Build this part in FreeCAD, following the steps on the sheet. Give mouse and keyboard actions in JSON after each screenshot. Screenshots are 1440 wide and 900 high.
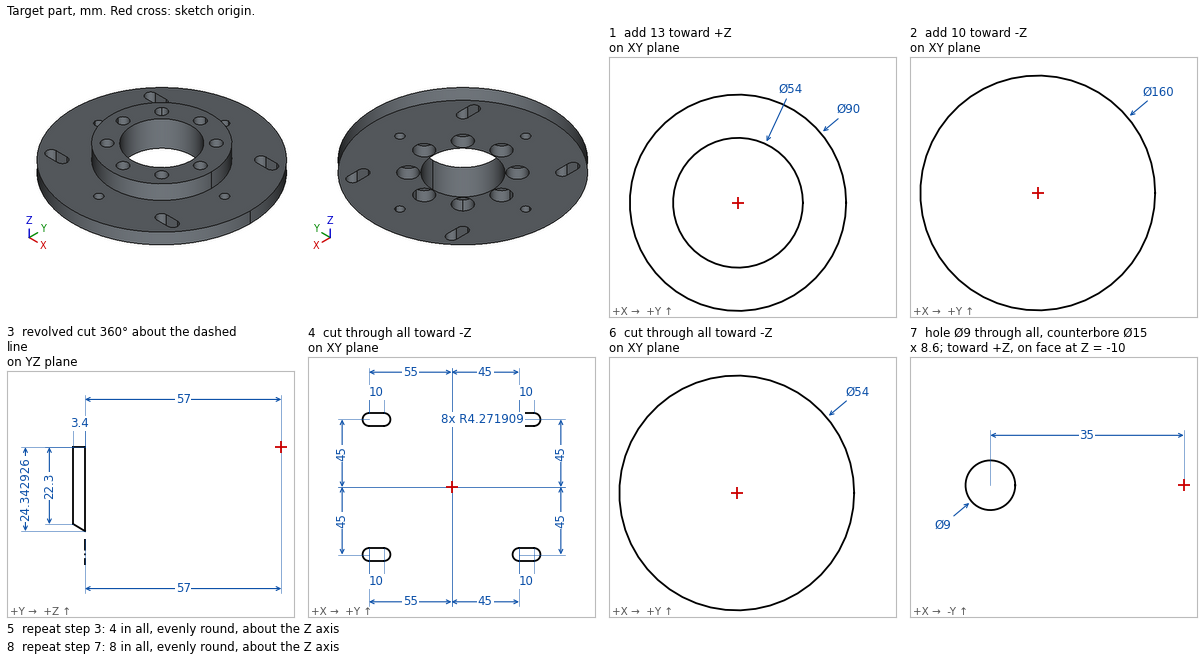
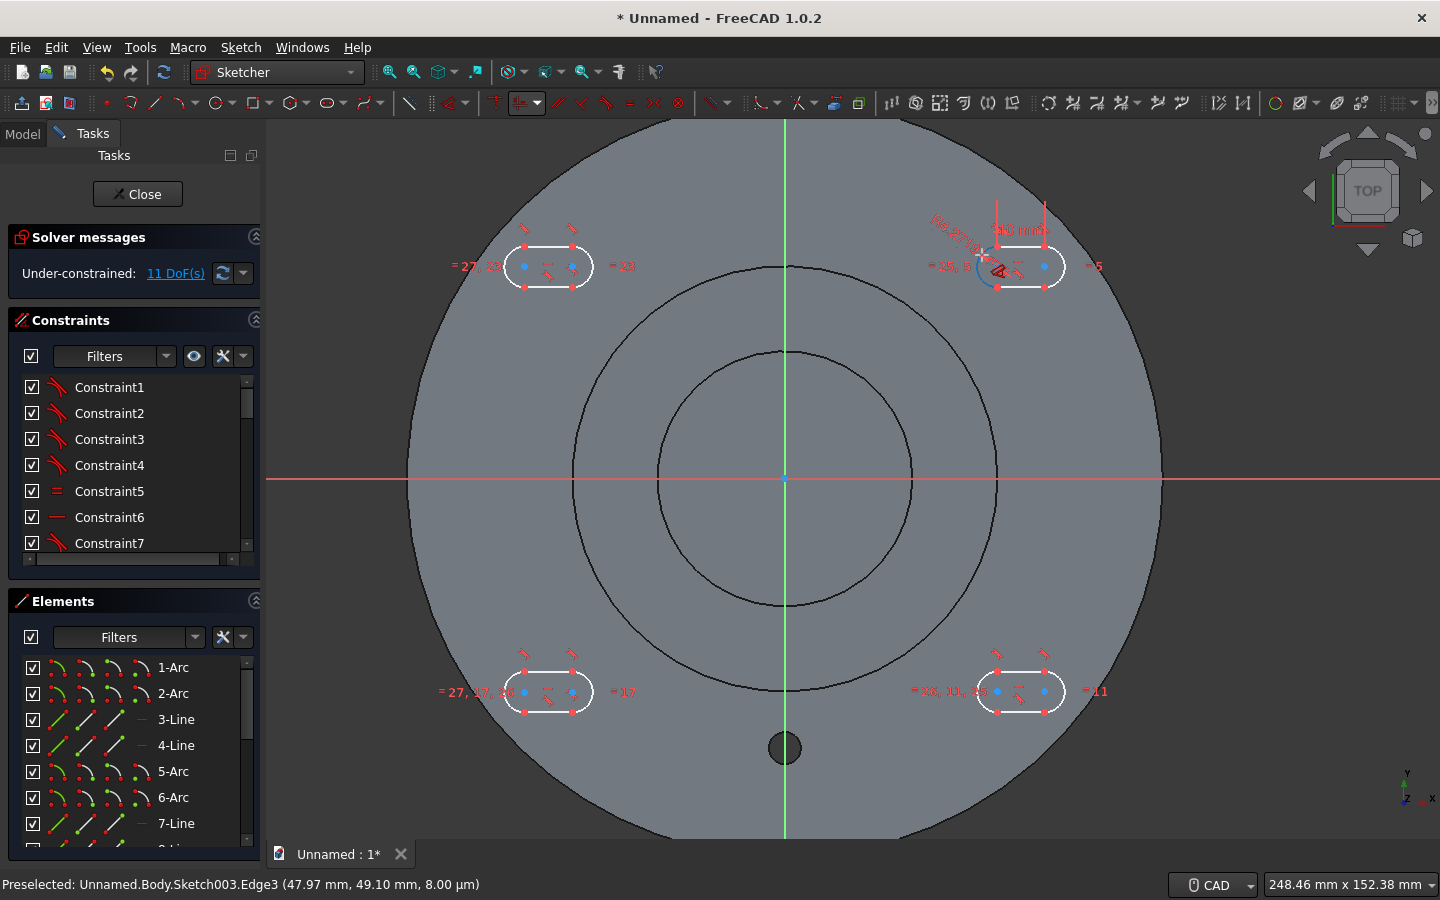
{"action": "left_click", "coordinate": [1012, 672]}
{"action": "left_click", "coordinate": [1021, 638]}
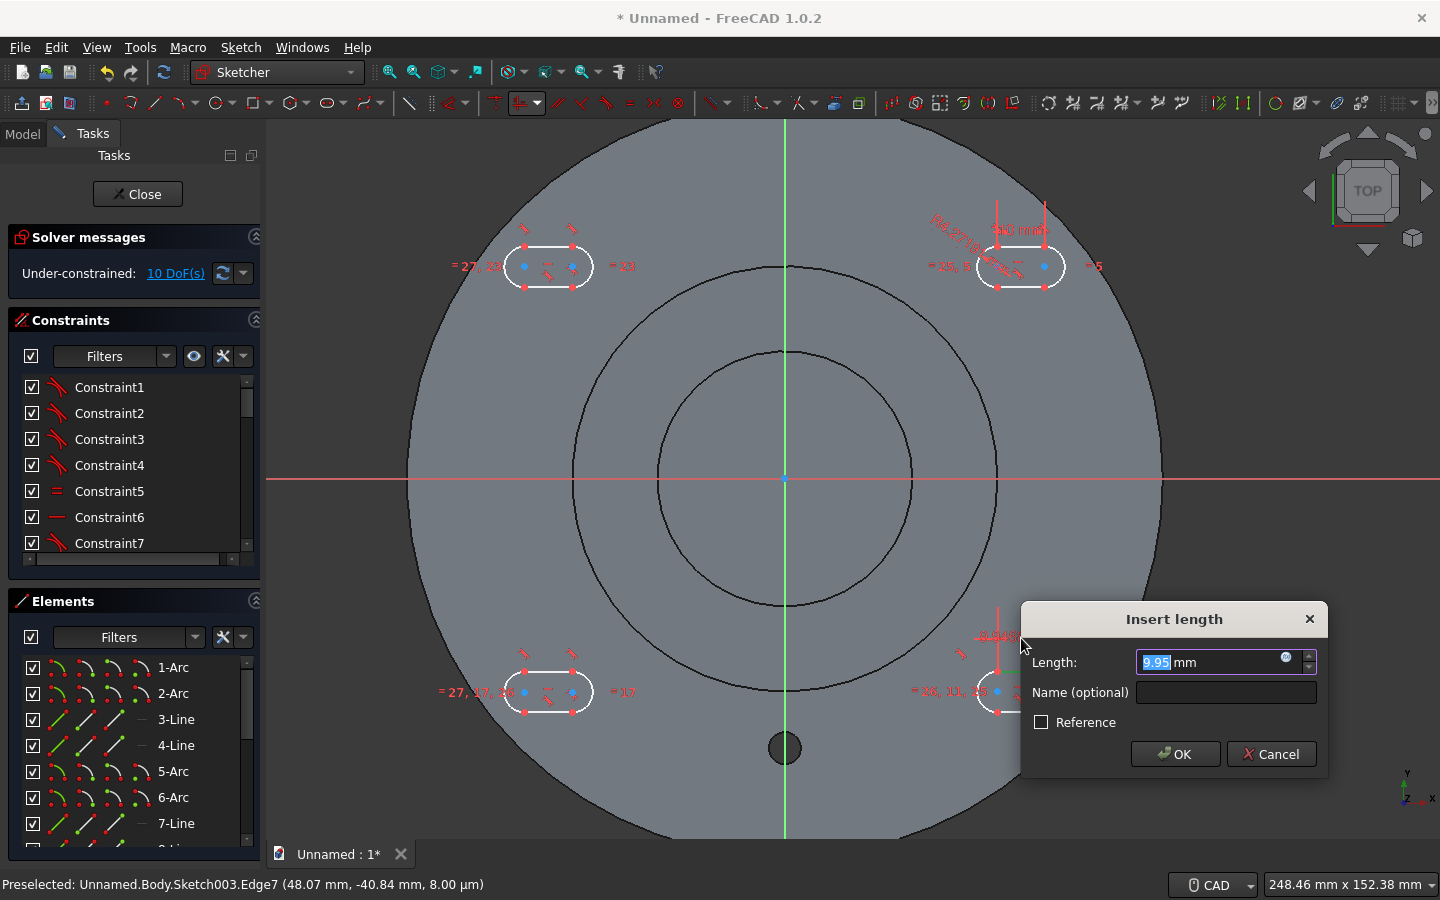
{"action": "type", "text": "10"}
{"action": "key", "text": "Return"}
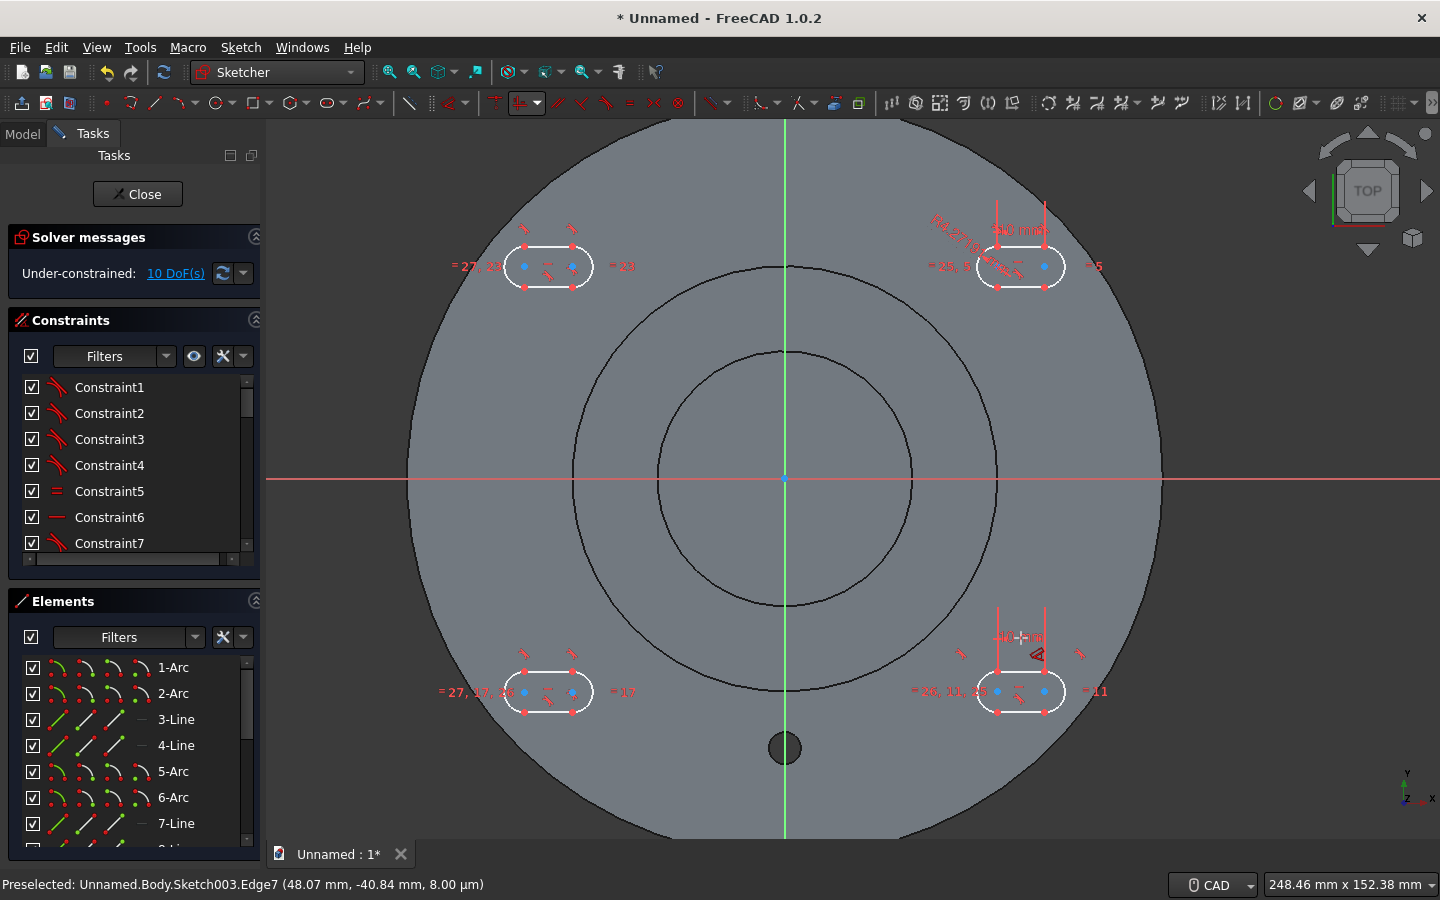
{"action": "left_click", "coordinate": [539, 672]}
{"action": "left_click", "coordinate": [549, 638]}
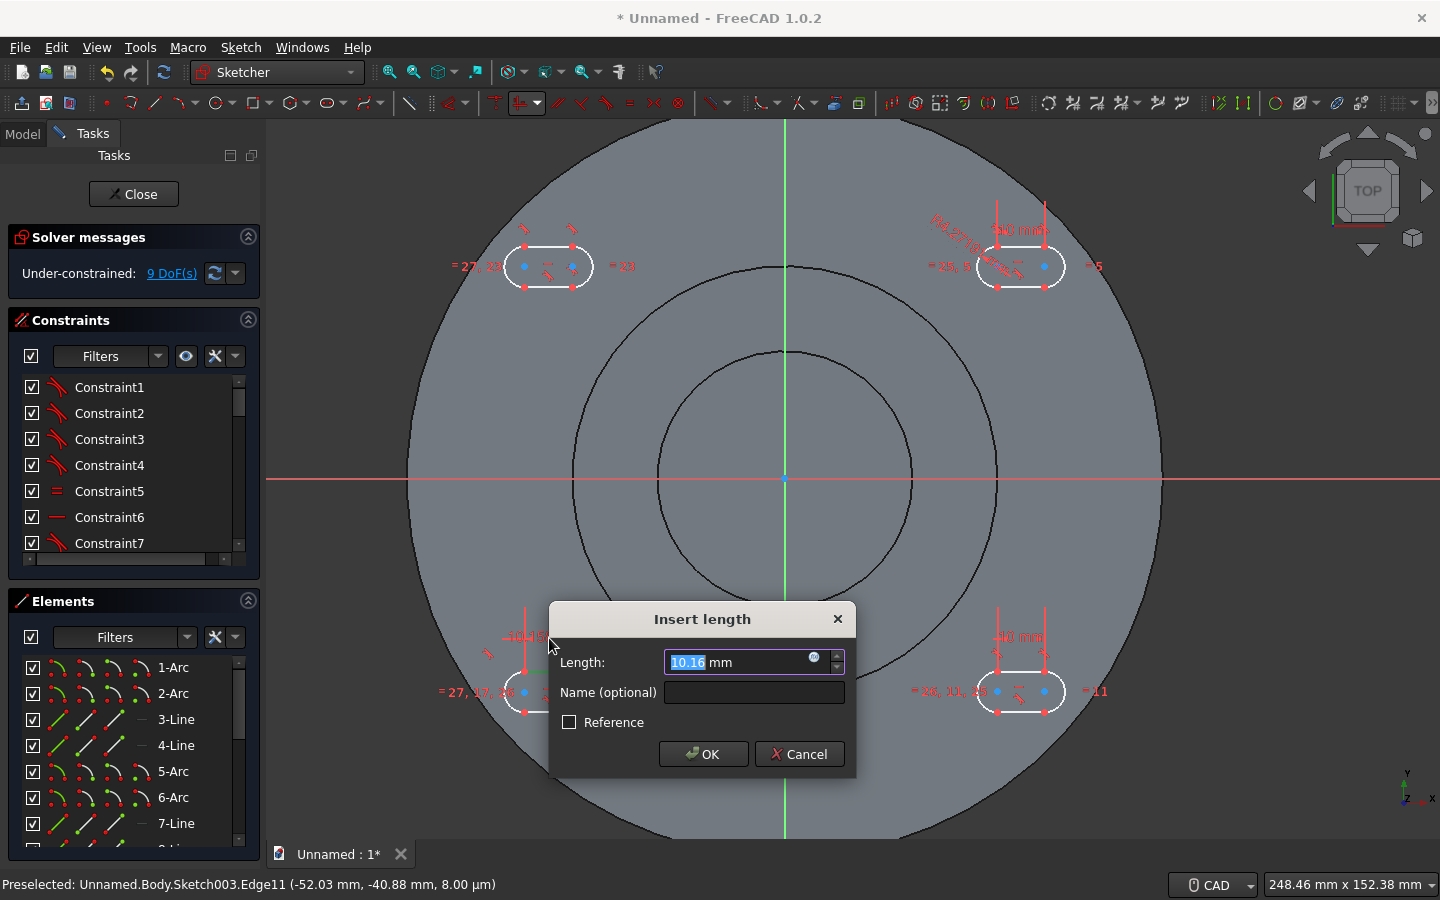
{"action": "type", "text": "10"}
{"action": "key", "text": "Return"}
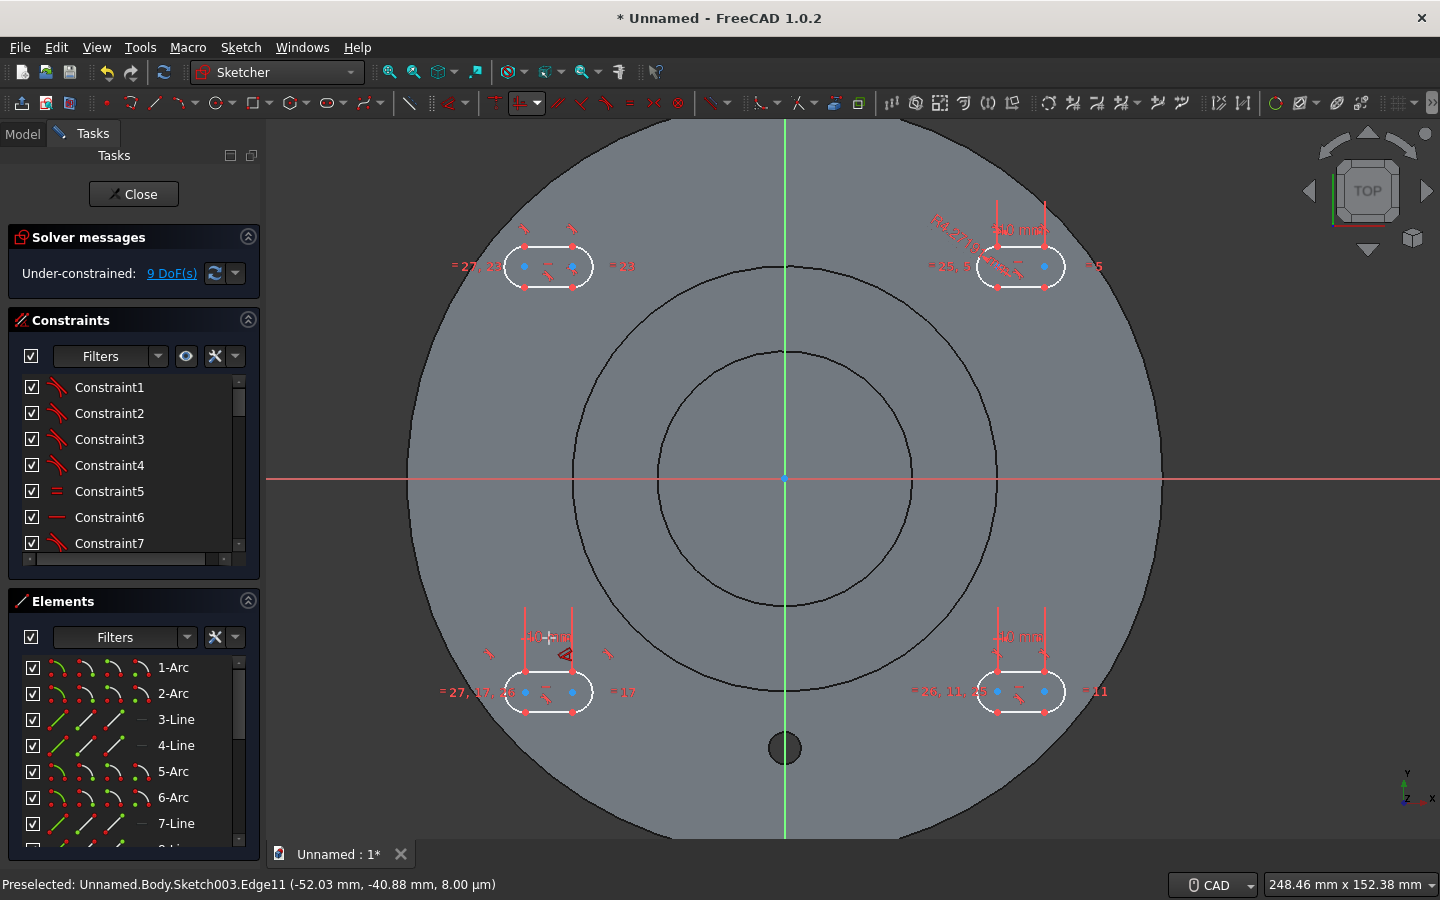
{"action": "left_click", "coordinate": [539, 247]}
{"action": "left_click", "coordinate": [549, 213]}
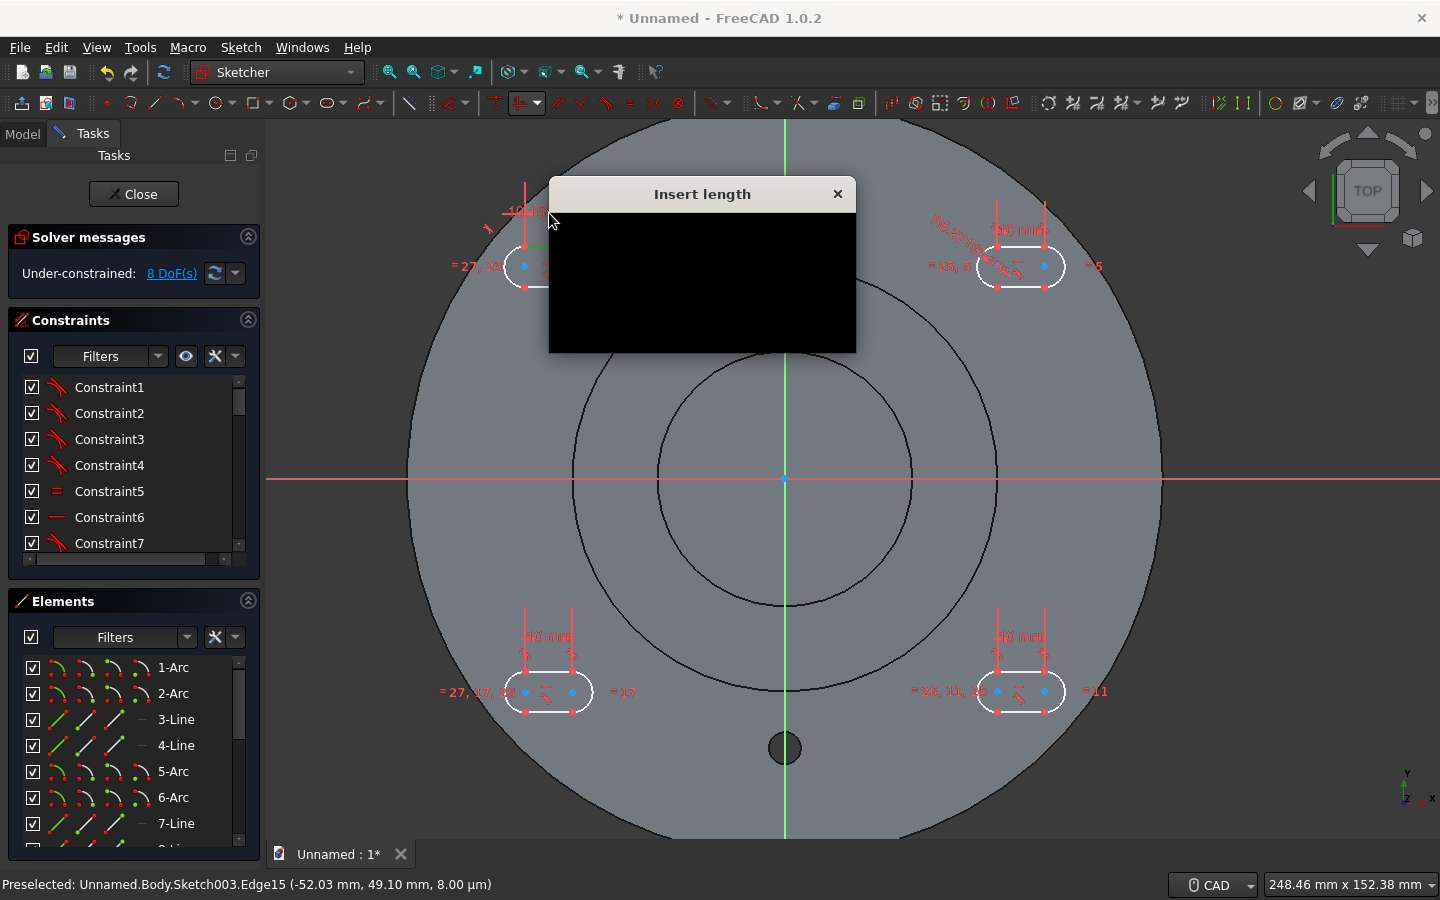
{"action": "type", "text": "10"}
{"action": "key", "text": "Return"}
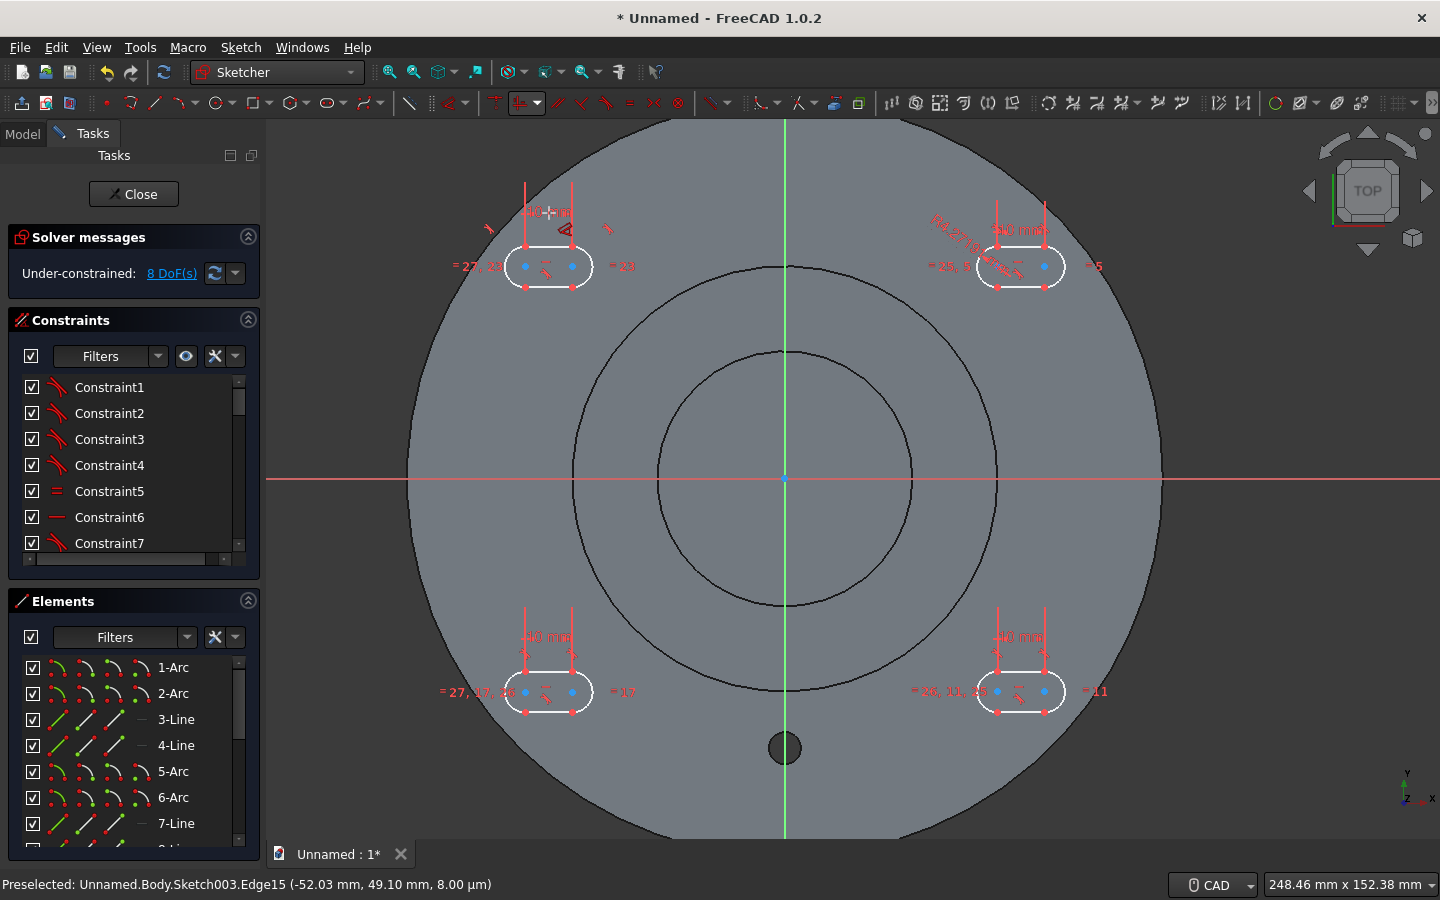
{"action": "left_click", "coordinate": [997, 247]}
{"action": "left_click", "coordinate": [891, 213]}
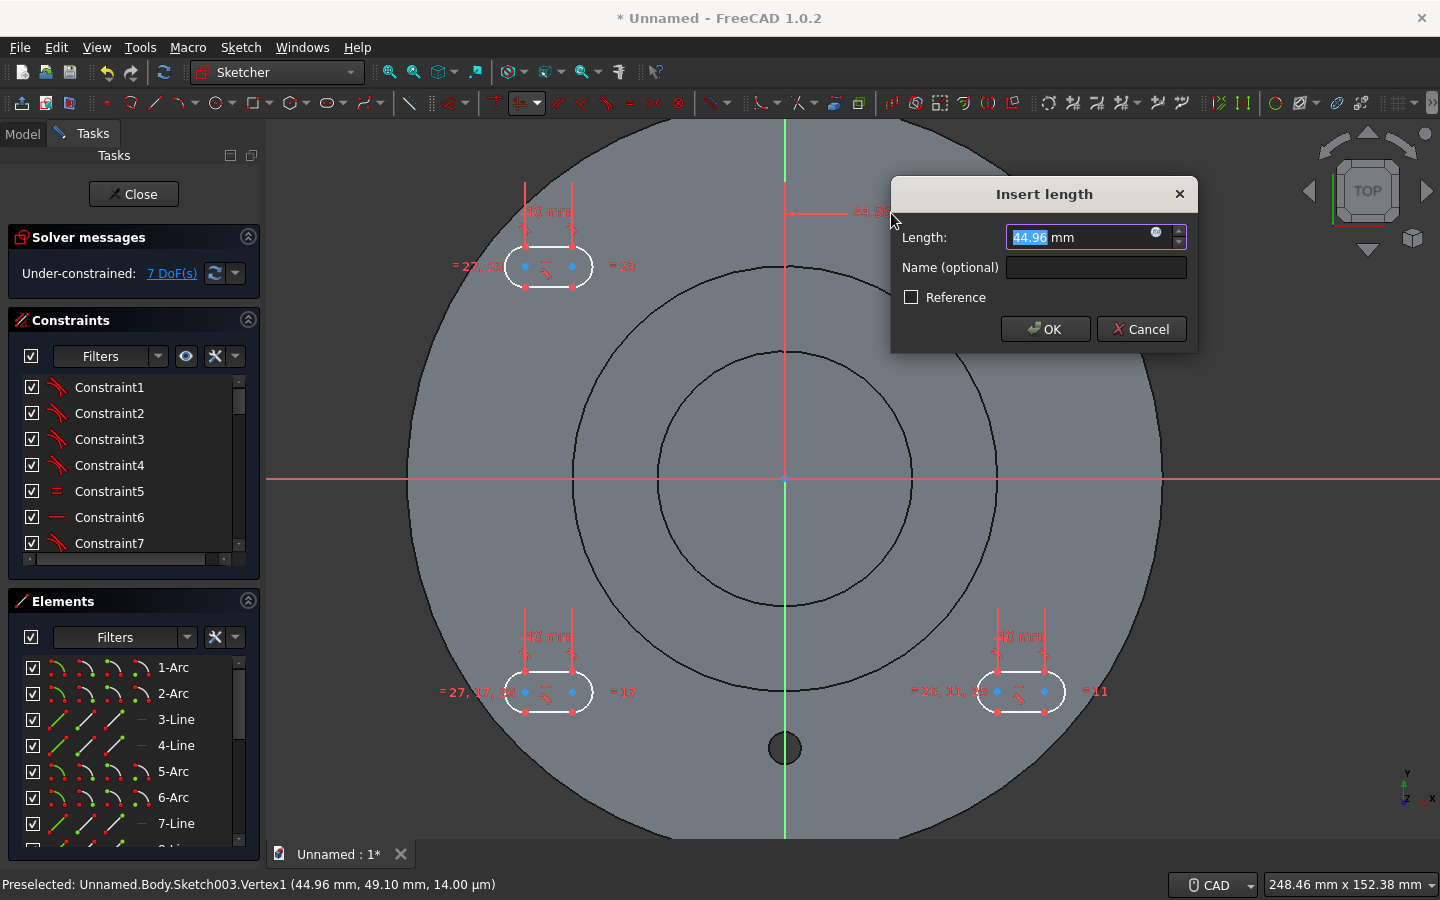
{"action": "type", "text": "45"}
{"action": "key", "text": "Return"}